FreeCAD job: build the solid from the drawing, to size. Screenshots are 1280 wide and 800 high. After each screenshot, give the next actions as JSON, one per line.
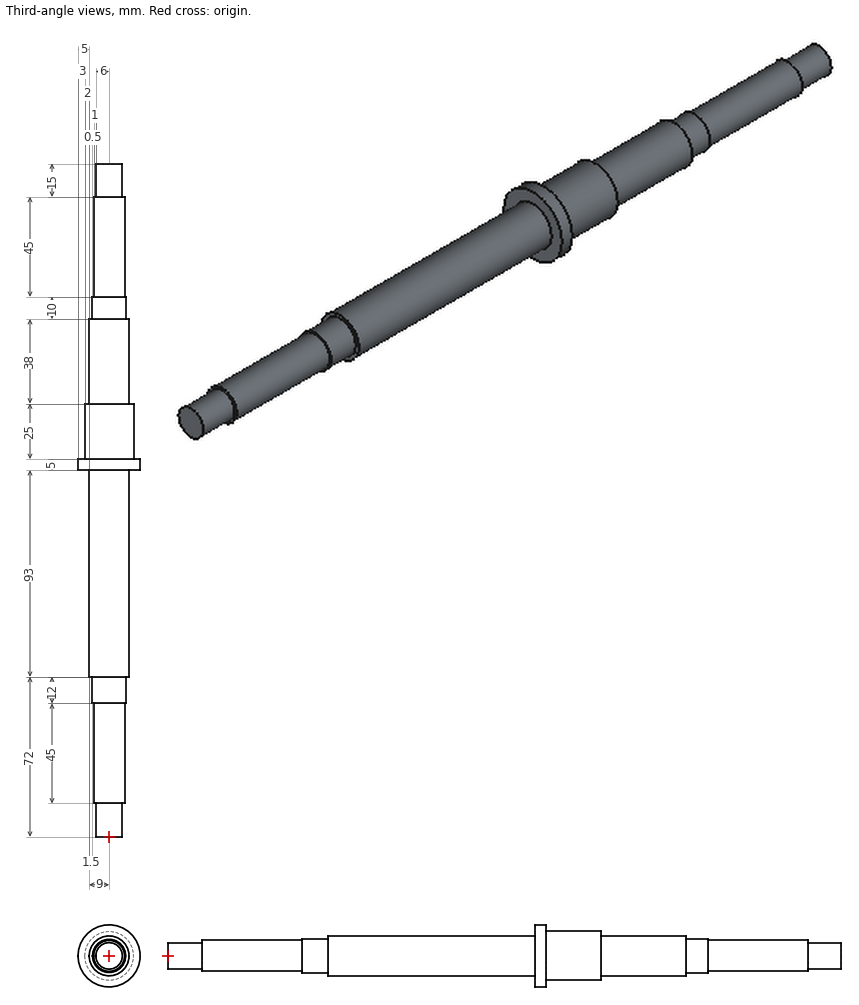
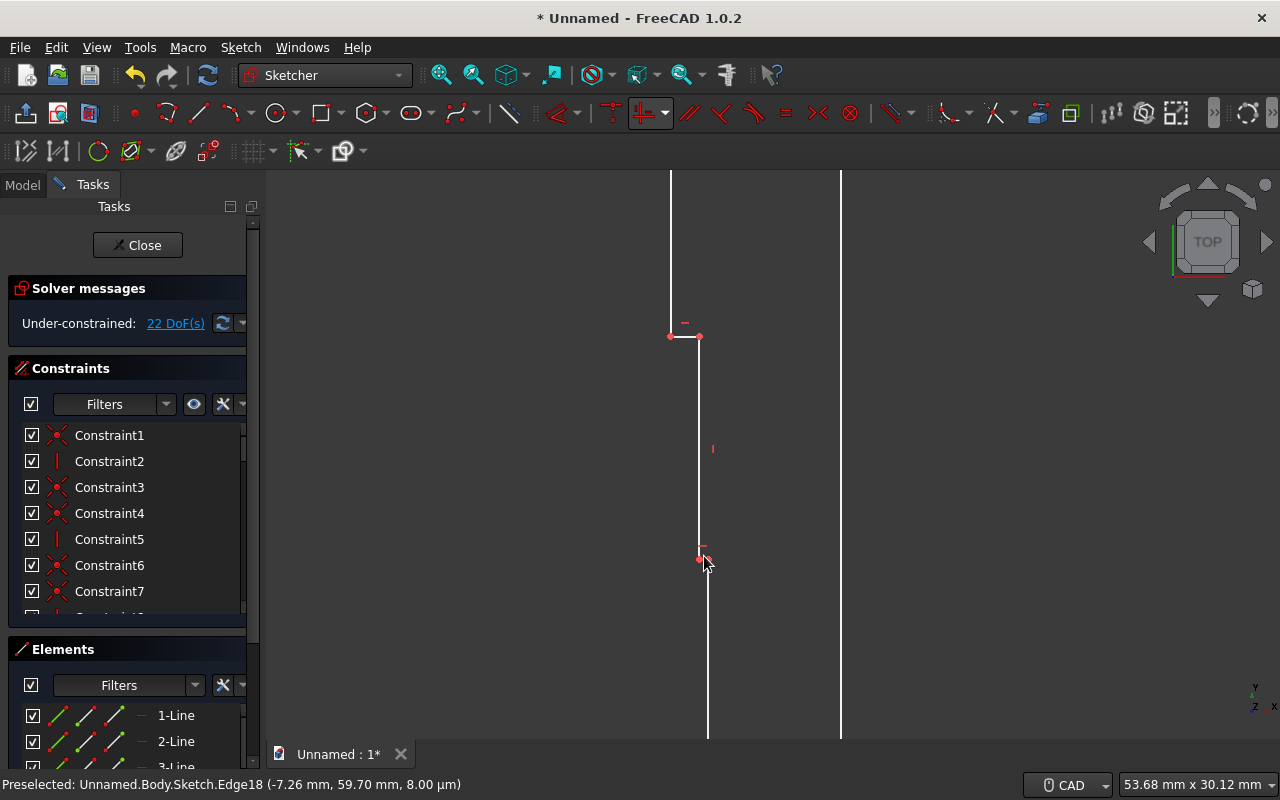
{"action": "scroll", "coordinate": [704, 560], "scroll_direction": "down", "scroll_amount": 14}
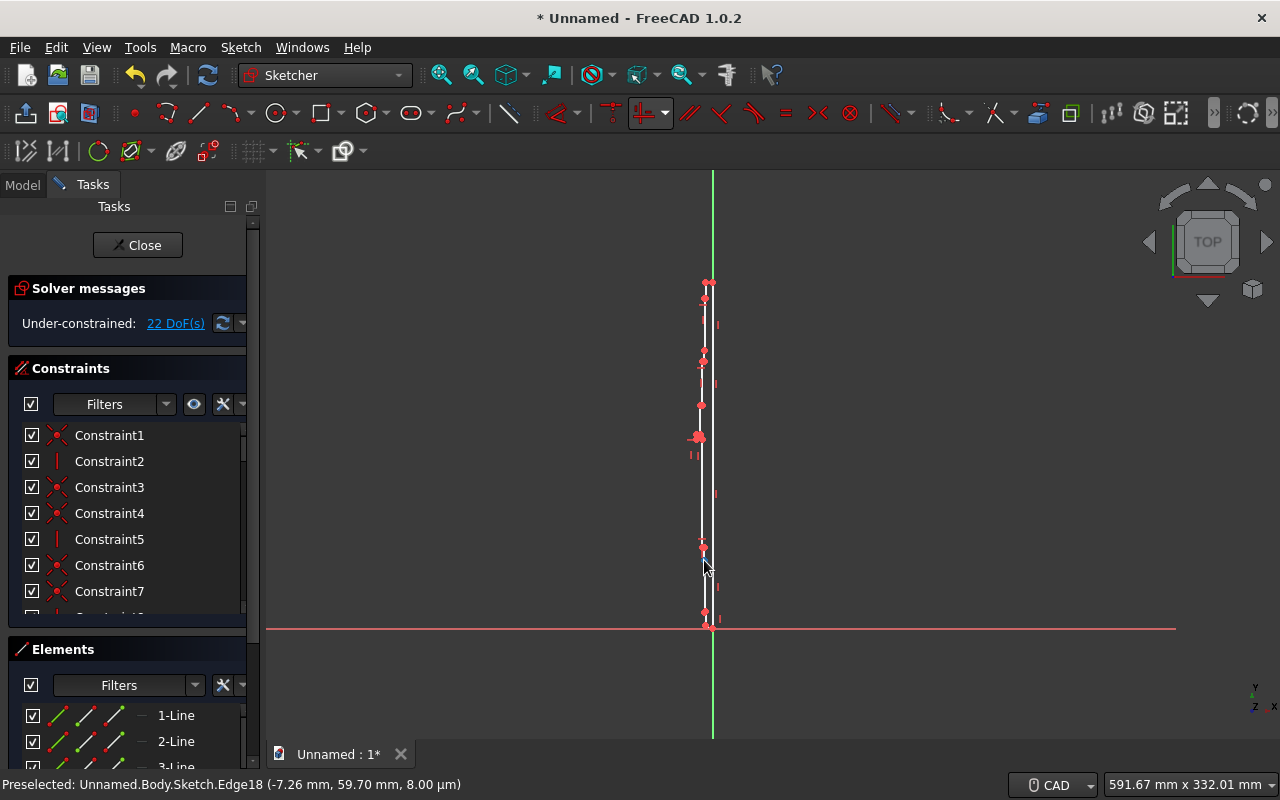
{"action": "scroll", "coordinate": [705, 612], "scroll_direction": "up", "scroll_amount": 14}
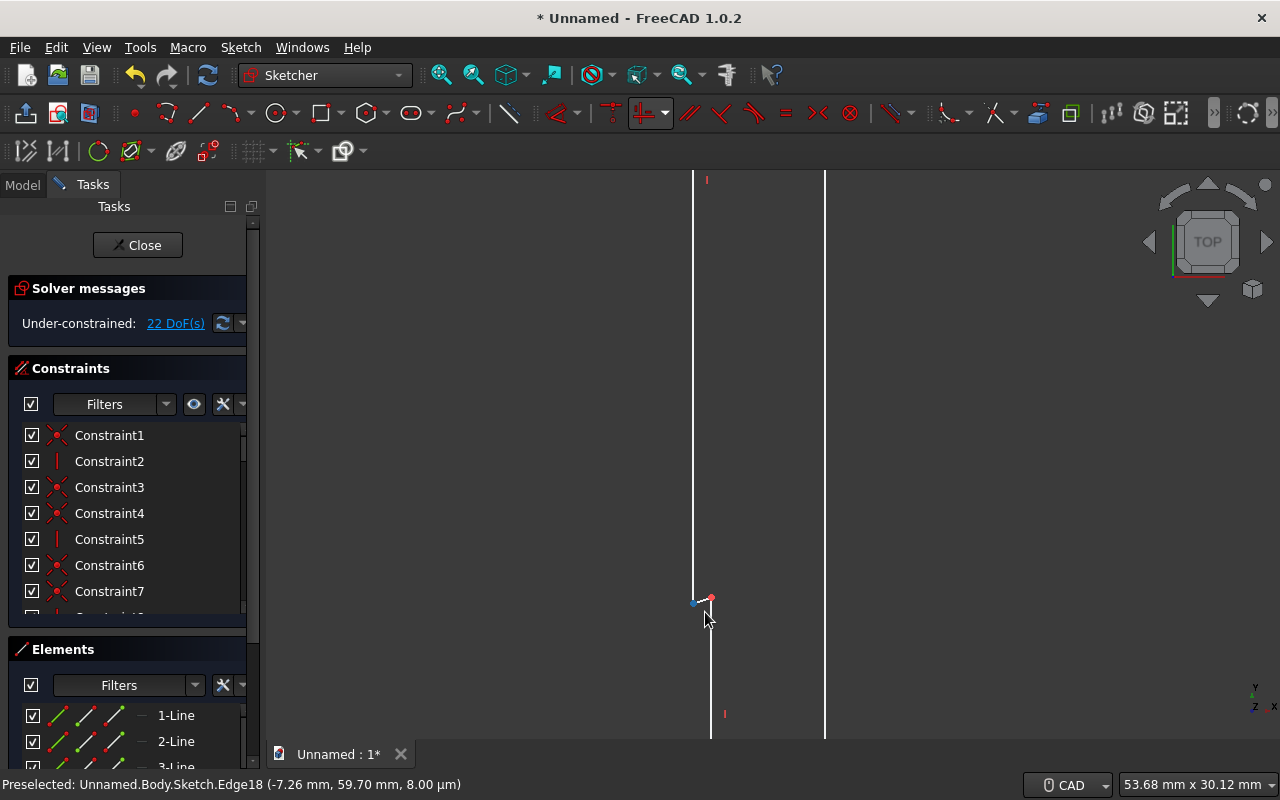
{"action": "left_click", "coordinate": [702, 601]}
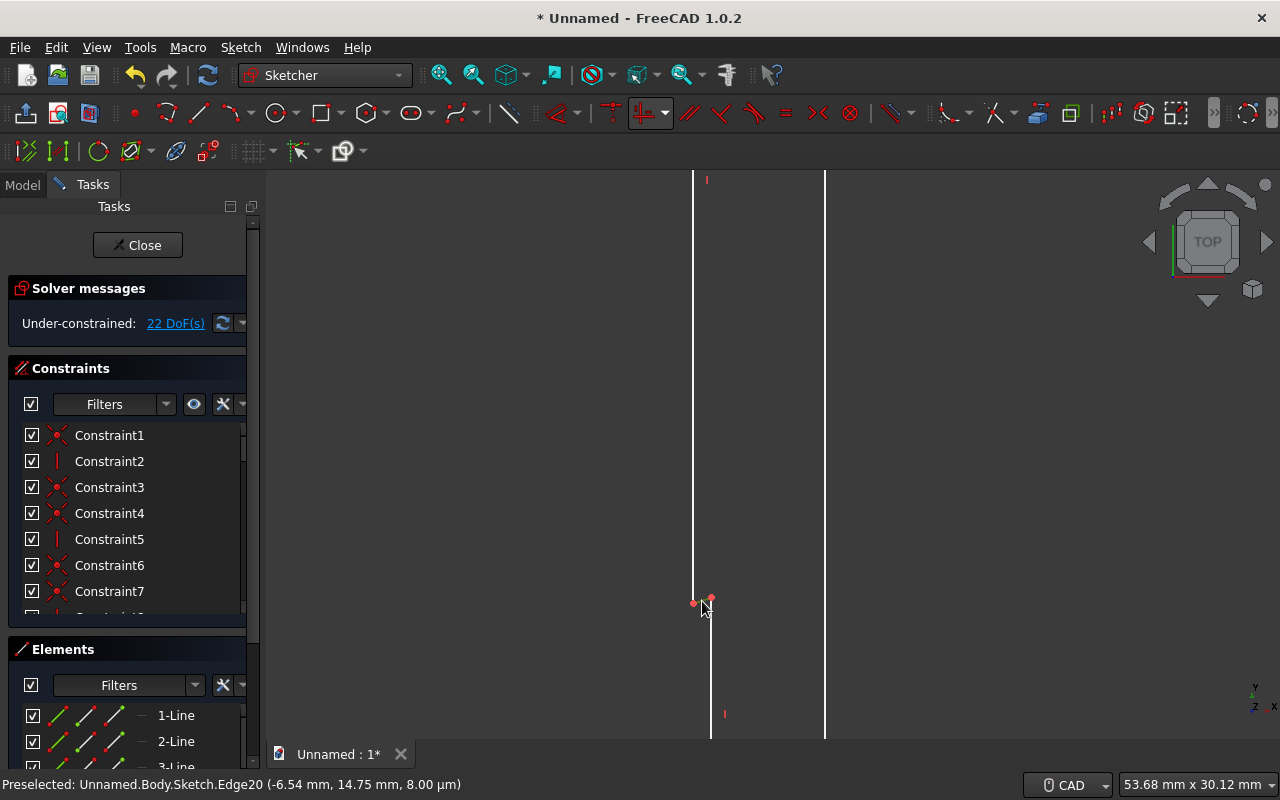
{"action": "key", "text": "h"}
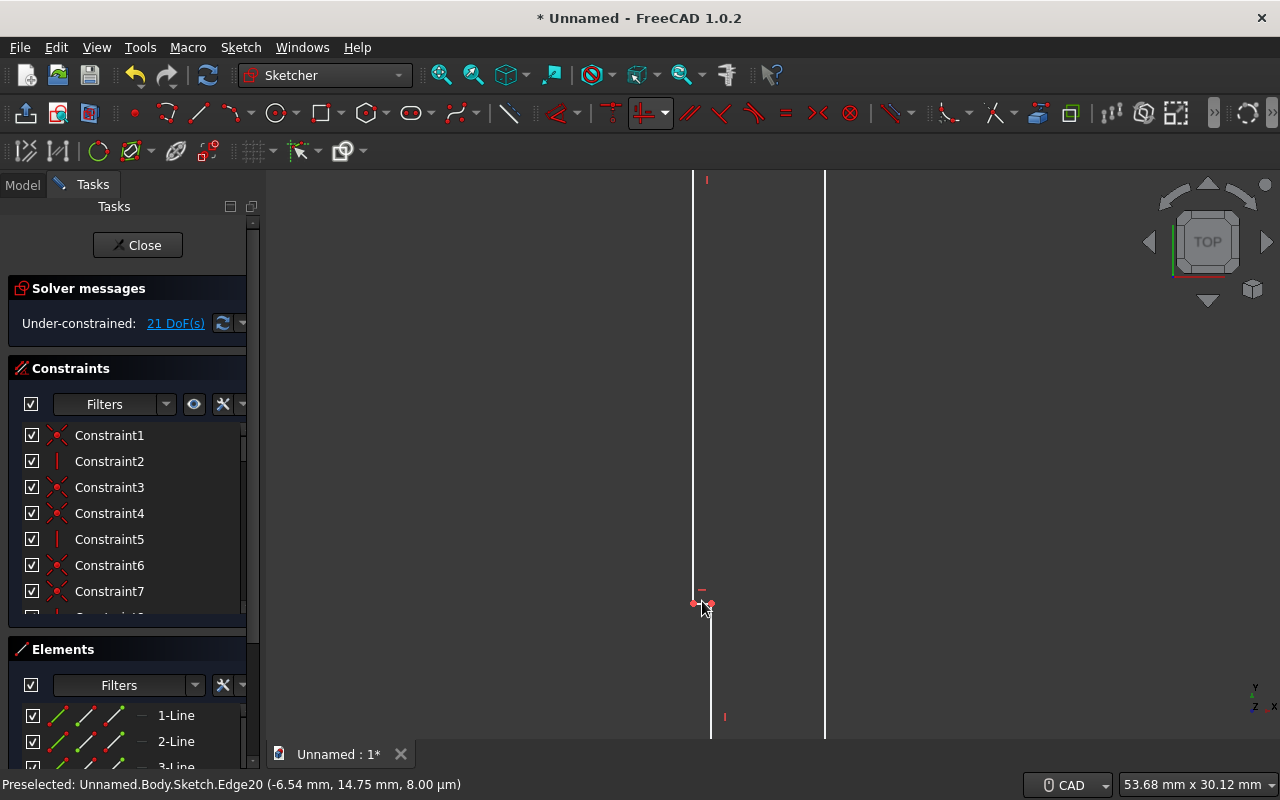
{"action": "scroll", "coordinate": [705, 612], "scroll_direction": "down", "scroll_amount": 14}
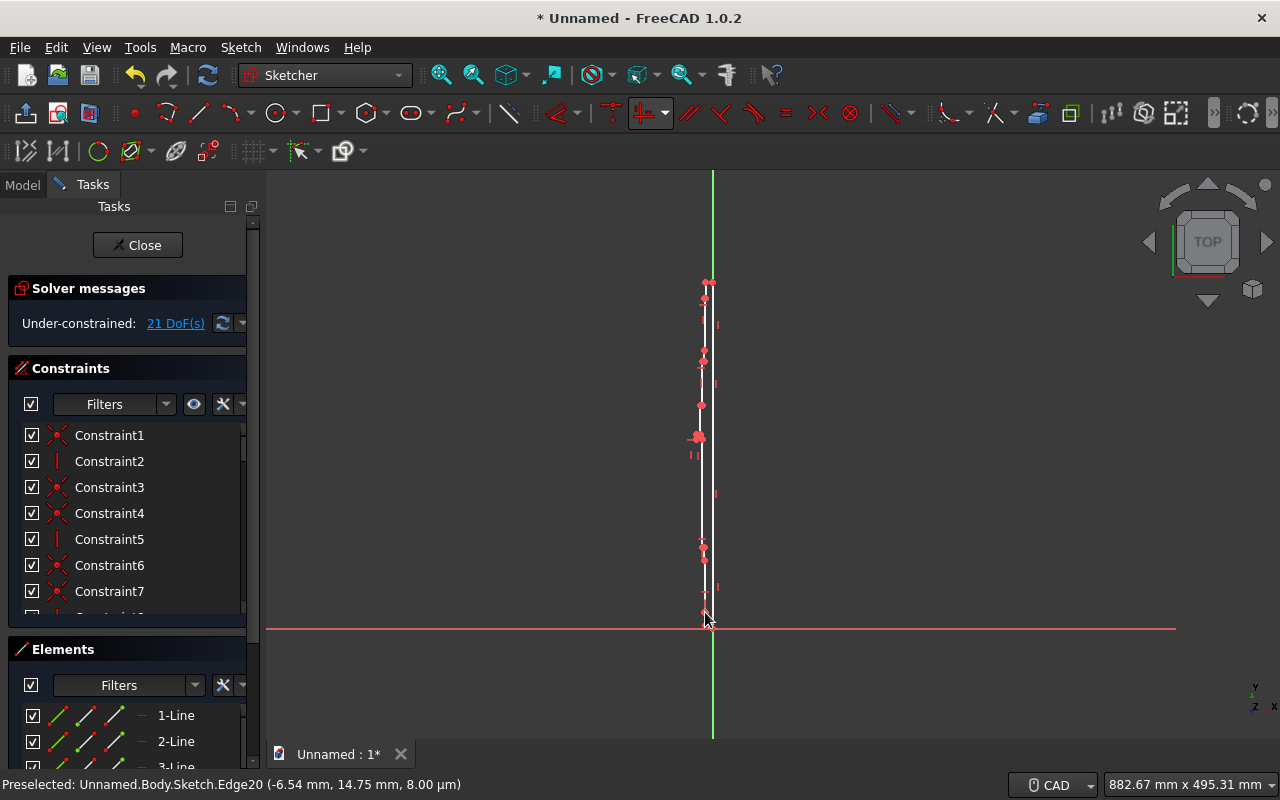
{"action": "scroll", "coordinate": [708, 627], "scroll_direction": "up", "scroll_amount": 10}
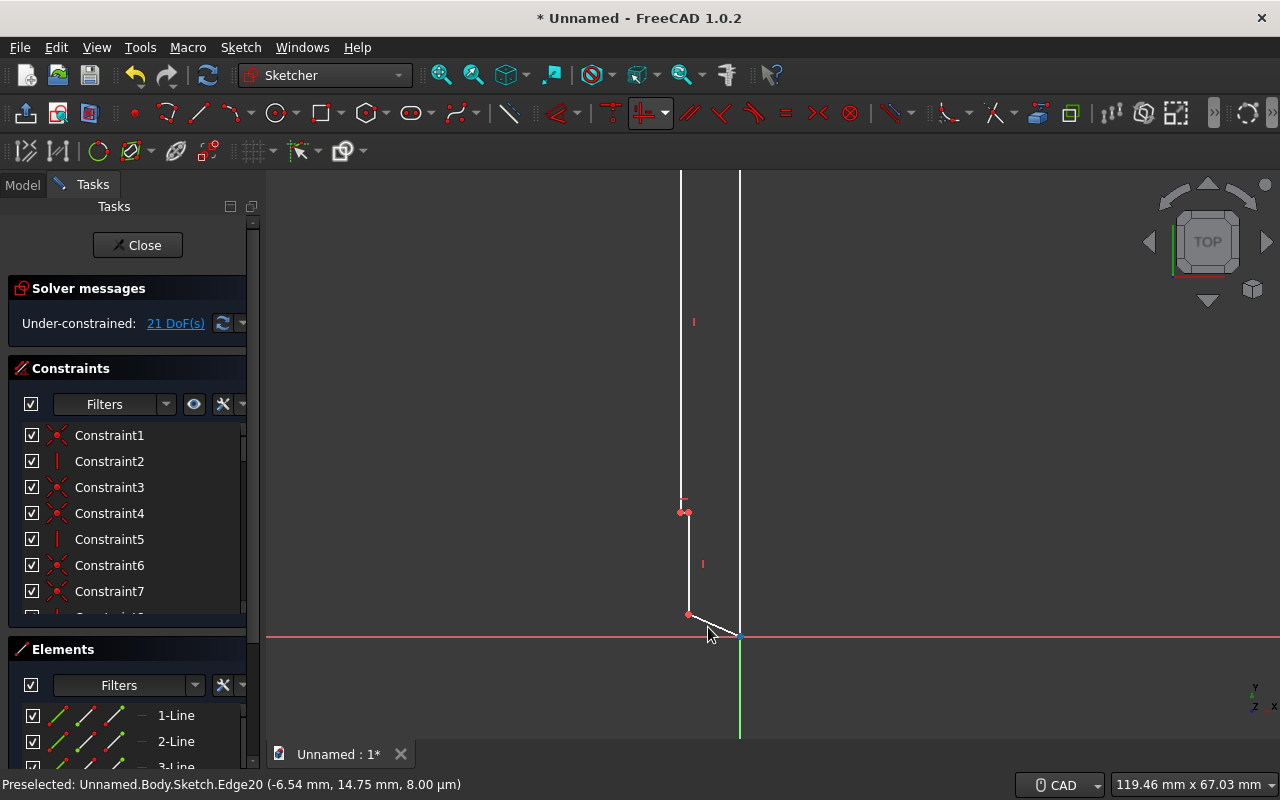
{"action": "left_click", "coordinate": [704, 621]}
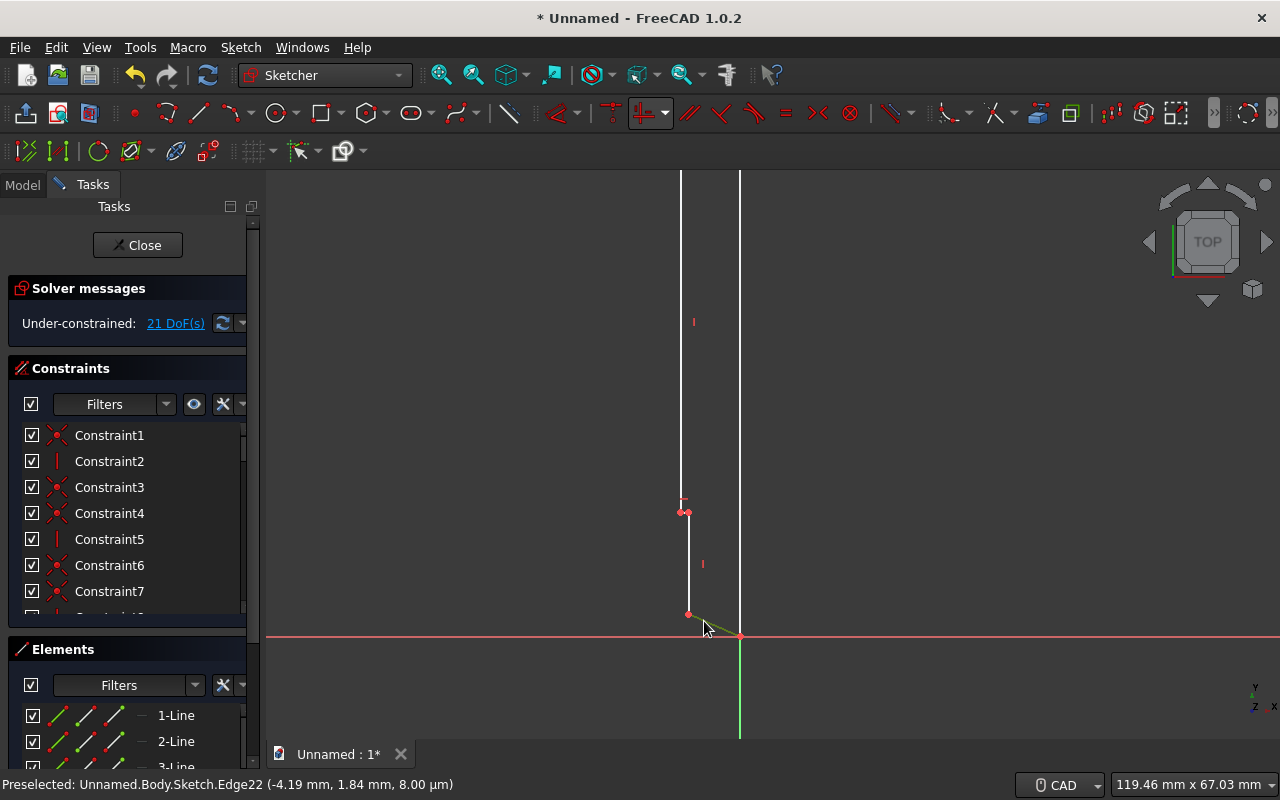
{"action": "key", "text": "h"}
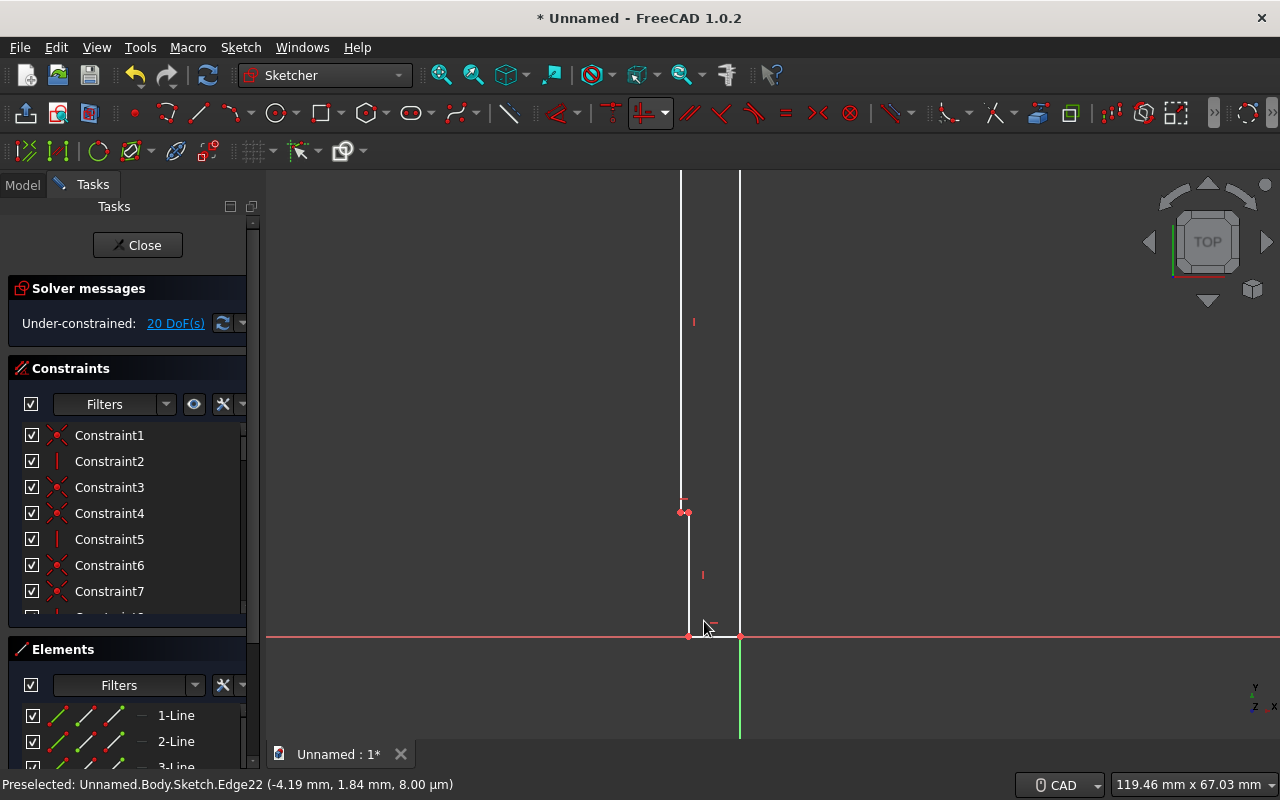
{"action": "key", "text": "d"}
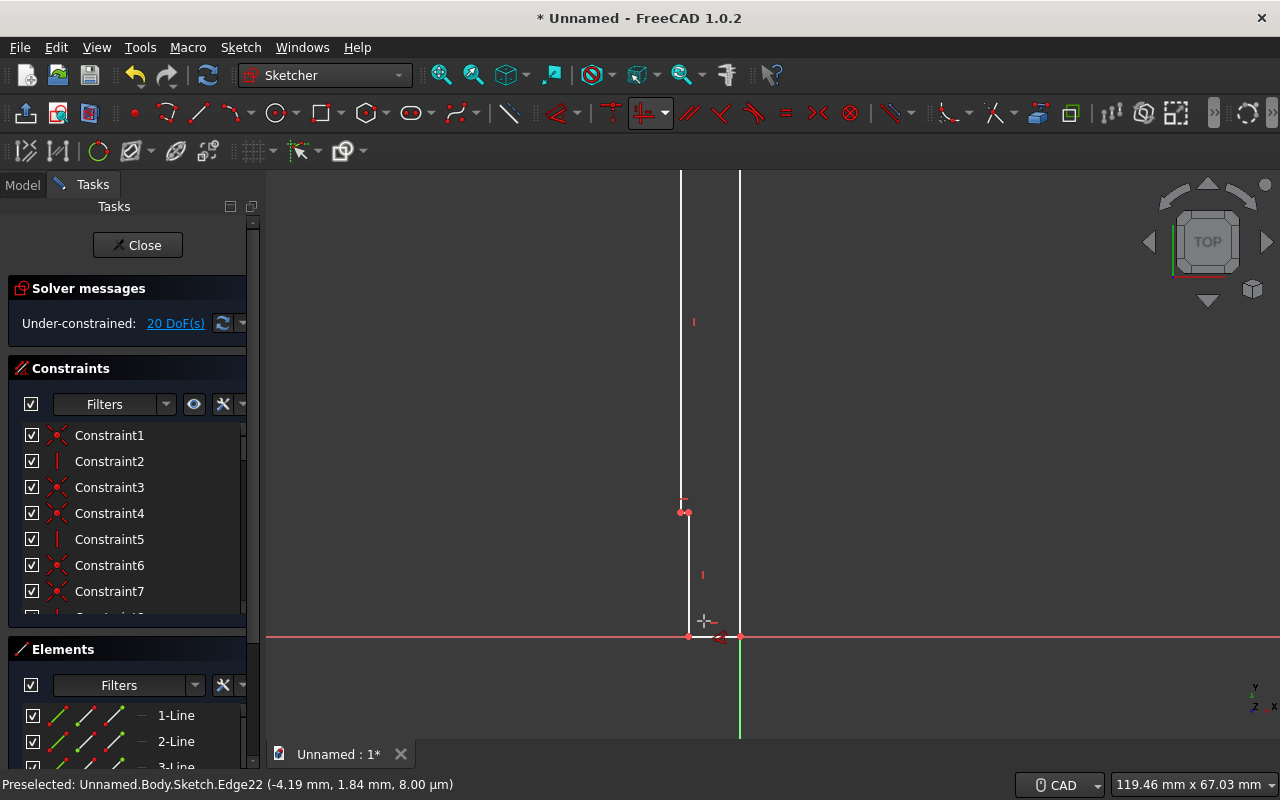
{"action": "scroll", "coordinate": [708, 627], "scroll_direction": "down", "scroll_amount": 10}